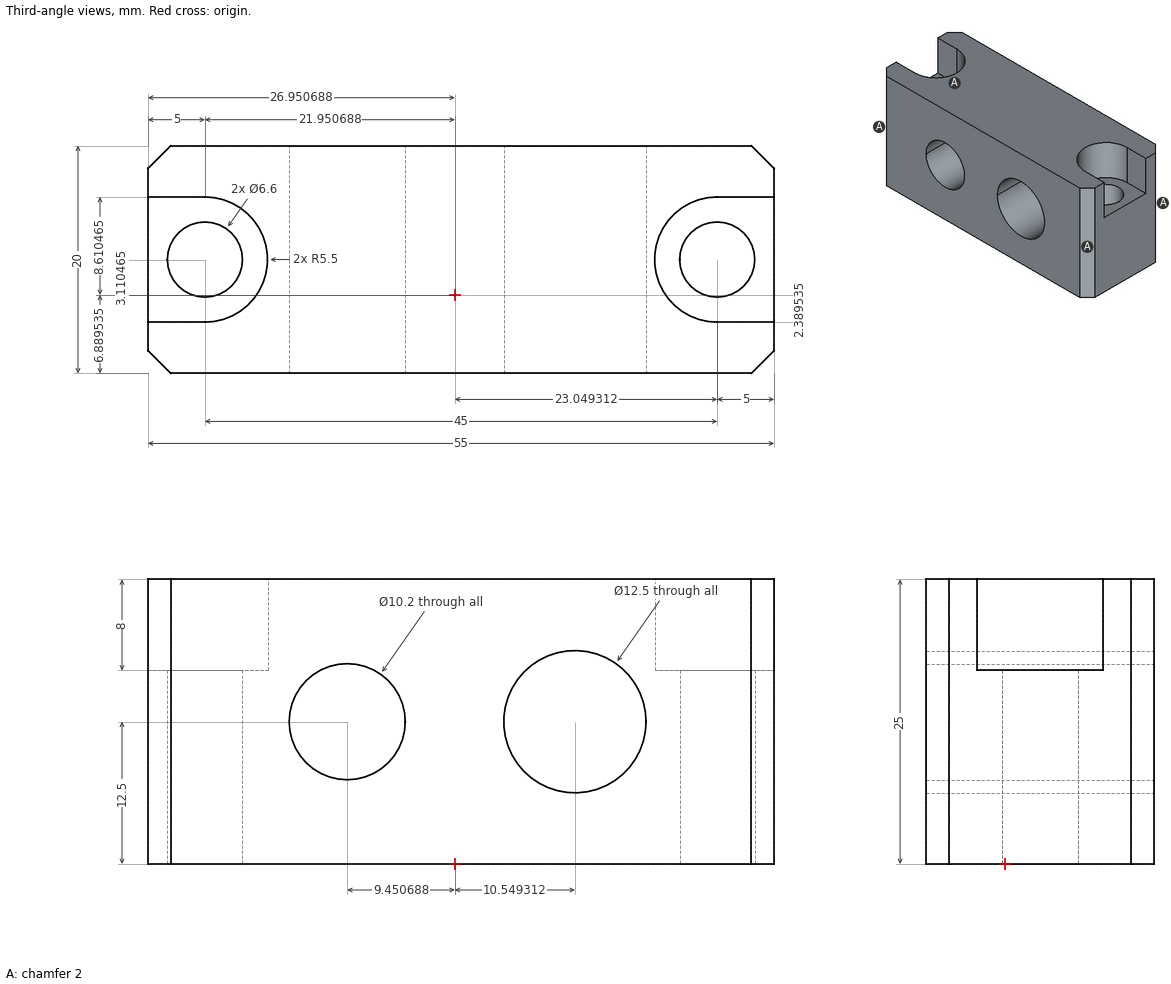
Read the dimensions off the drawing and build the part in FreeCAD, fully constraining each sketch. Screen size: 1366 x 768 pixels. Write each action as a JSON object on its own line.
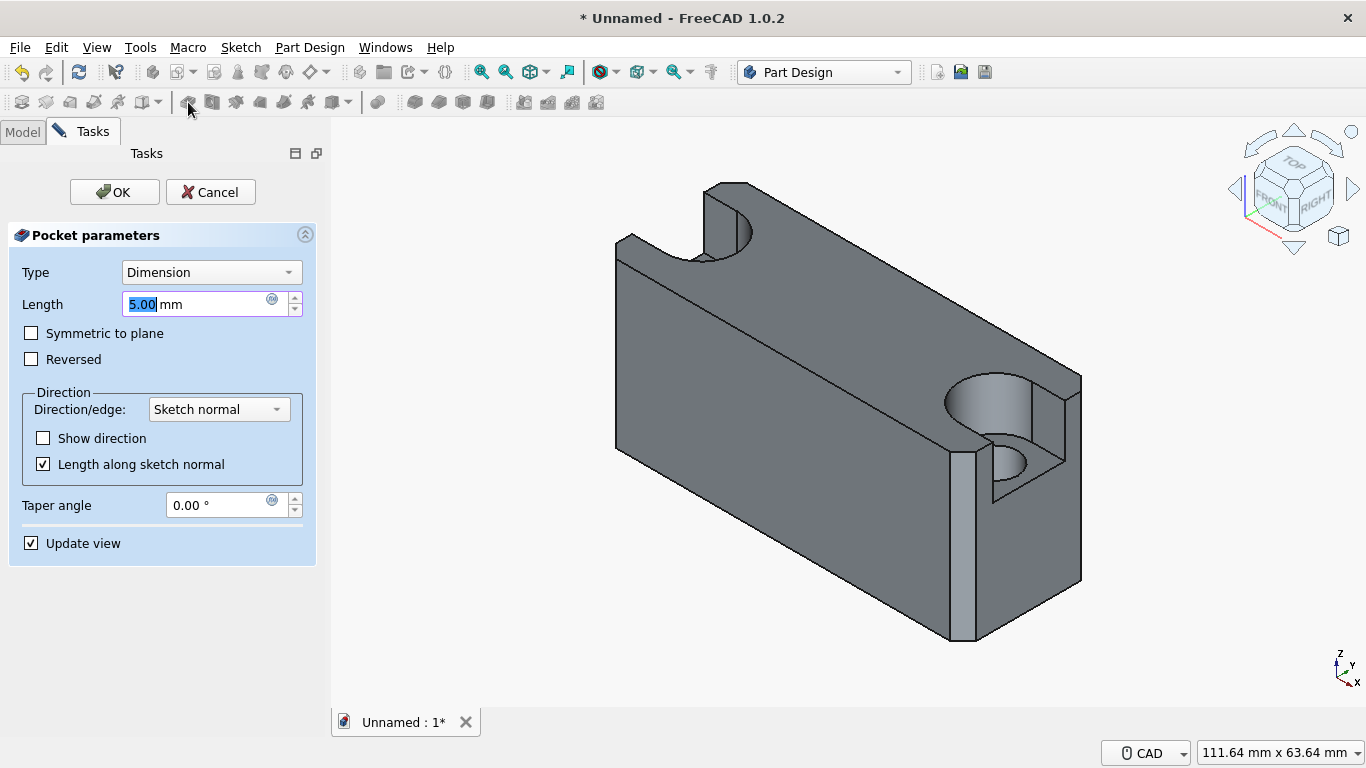
{"action": "left_click", "coordinate": [212, 272]}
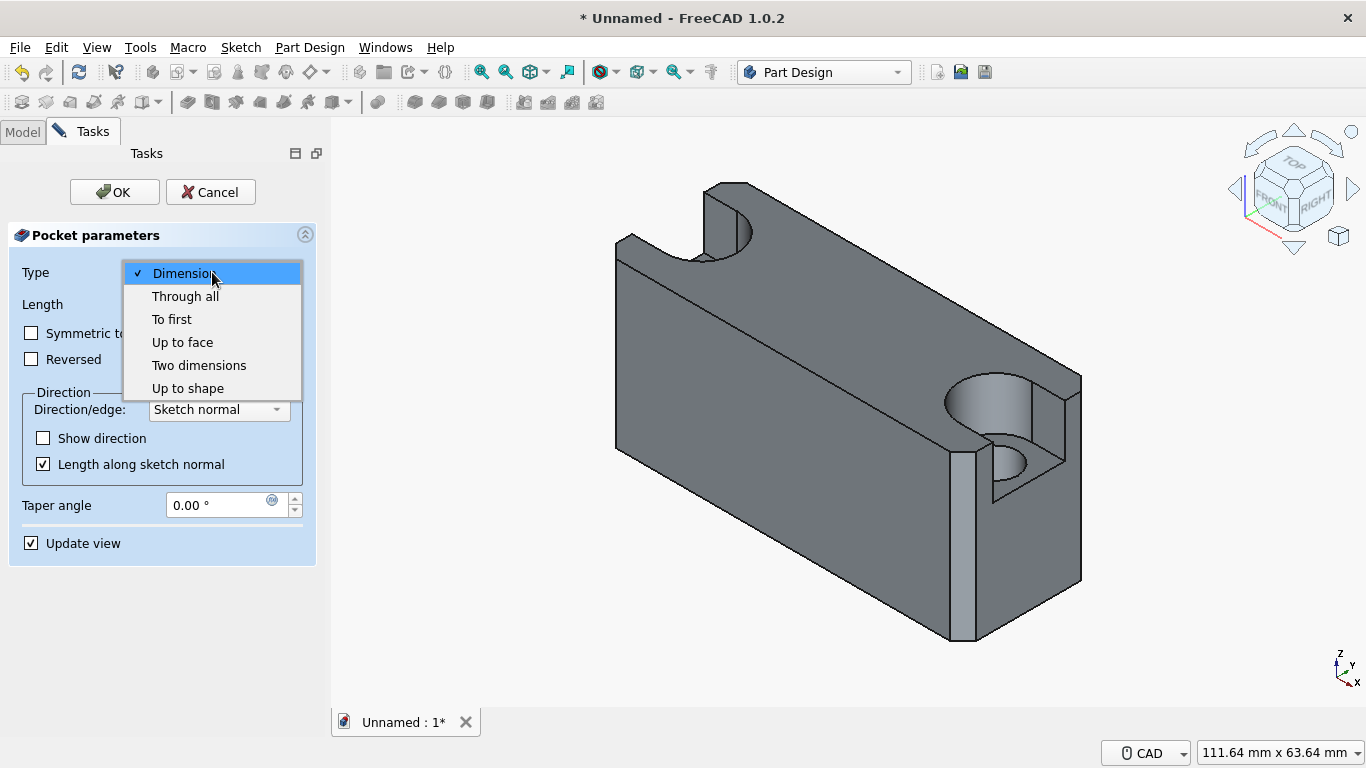
{"action": "left_click", "coordinate": [212, 296]}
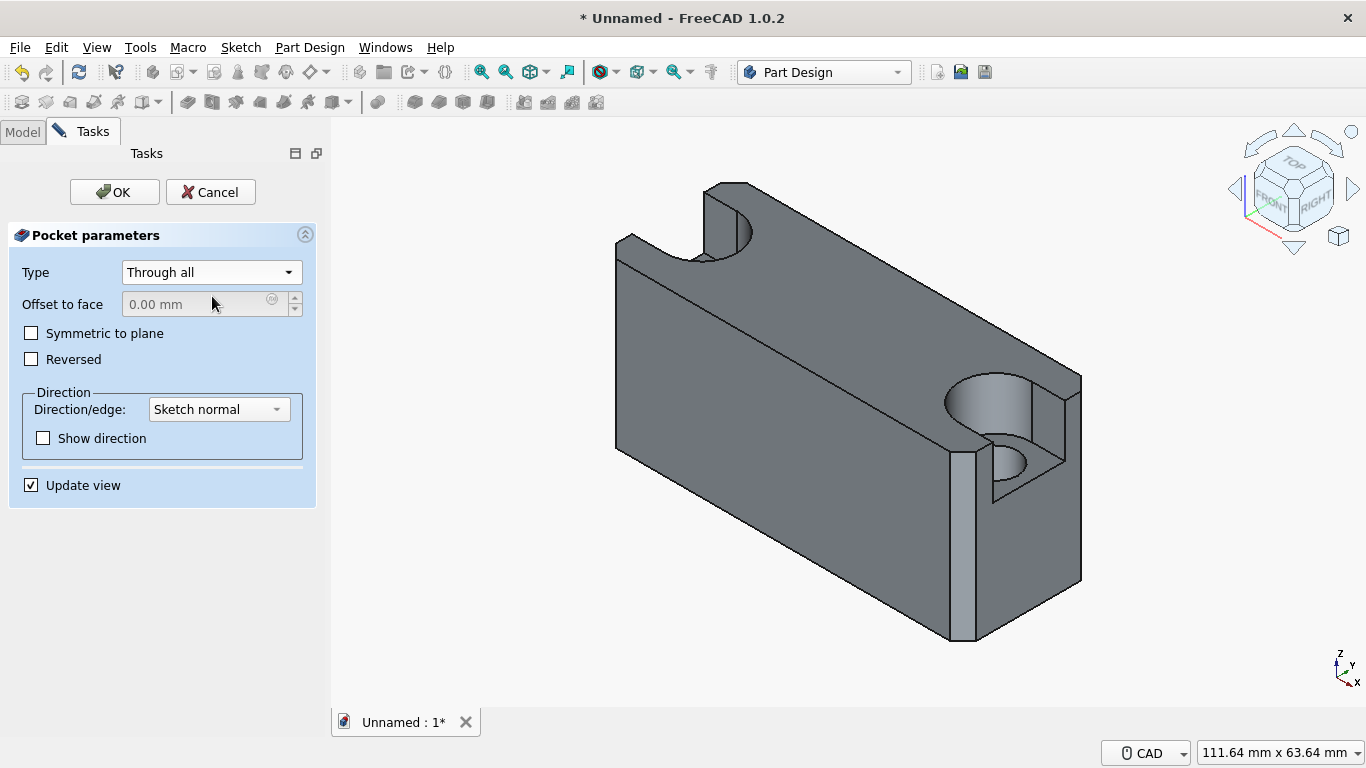
{"action": "left_click", "coordinate": [115, 192]}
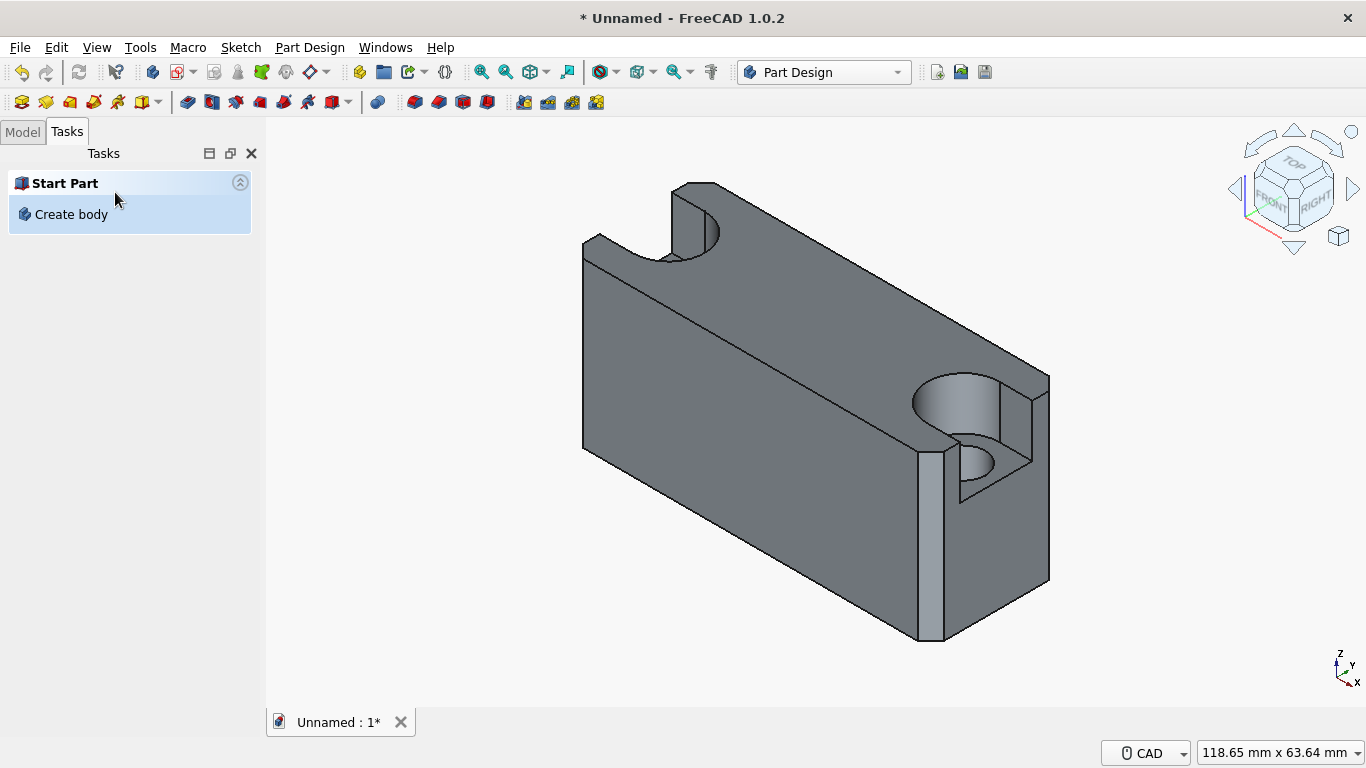
{"action": "left_click", "coordinate": [798, 476]}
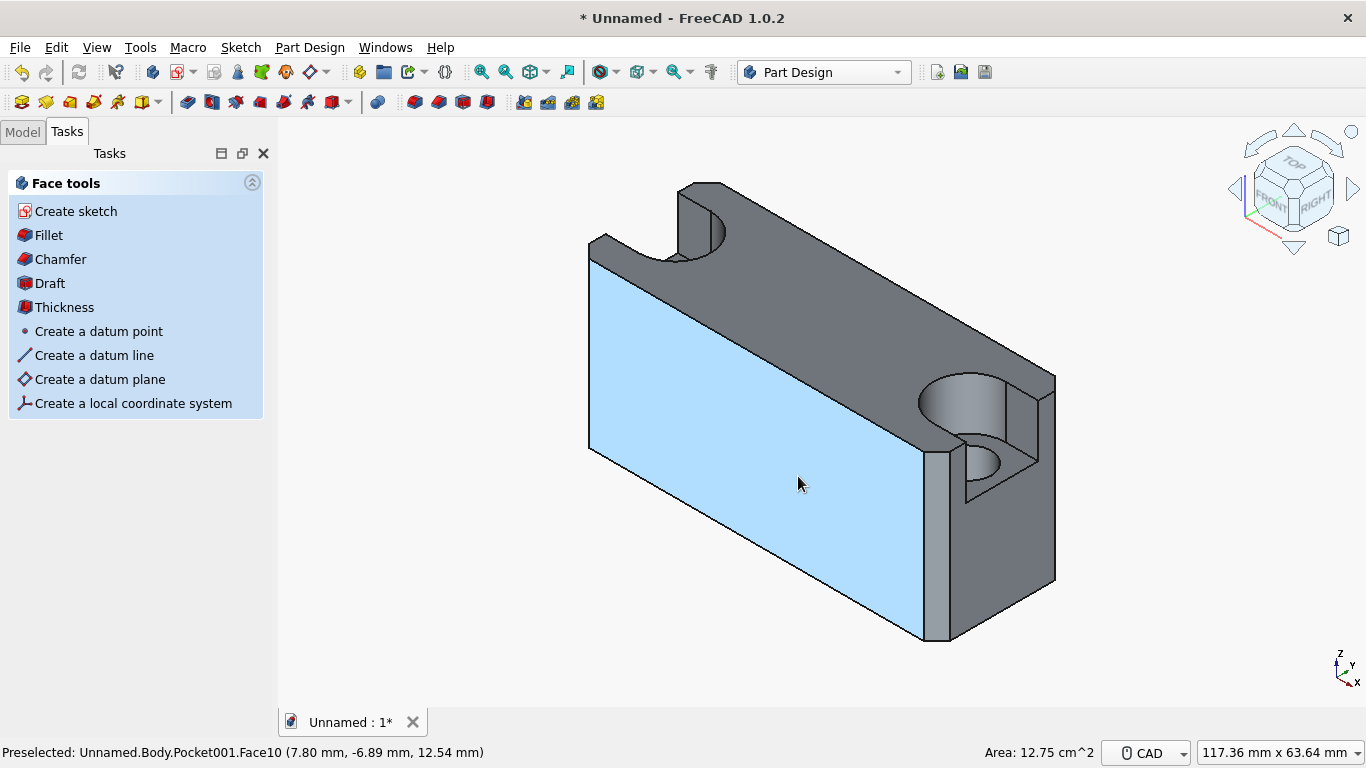
{"action": "left_click", "coordinate": [178, 72]}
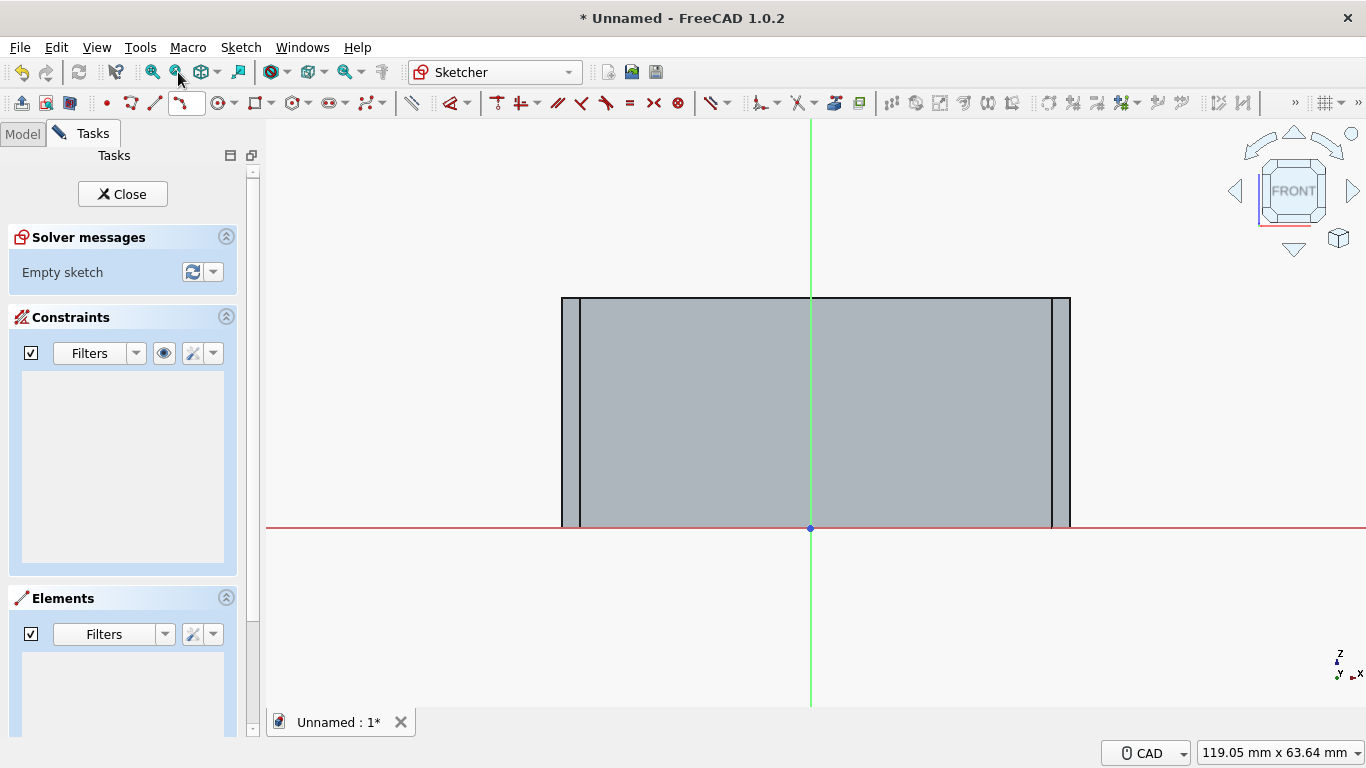
{"action": "scroll", "coordinate": [741, 475], "scroll_direction": "up", "scroll_amount": 4}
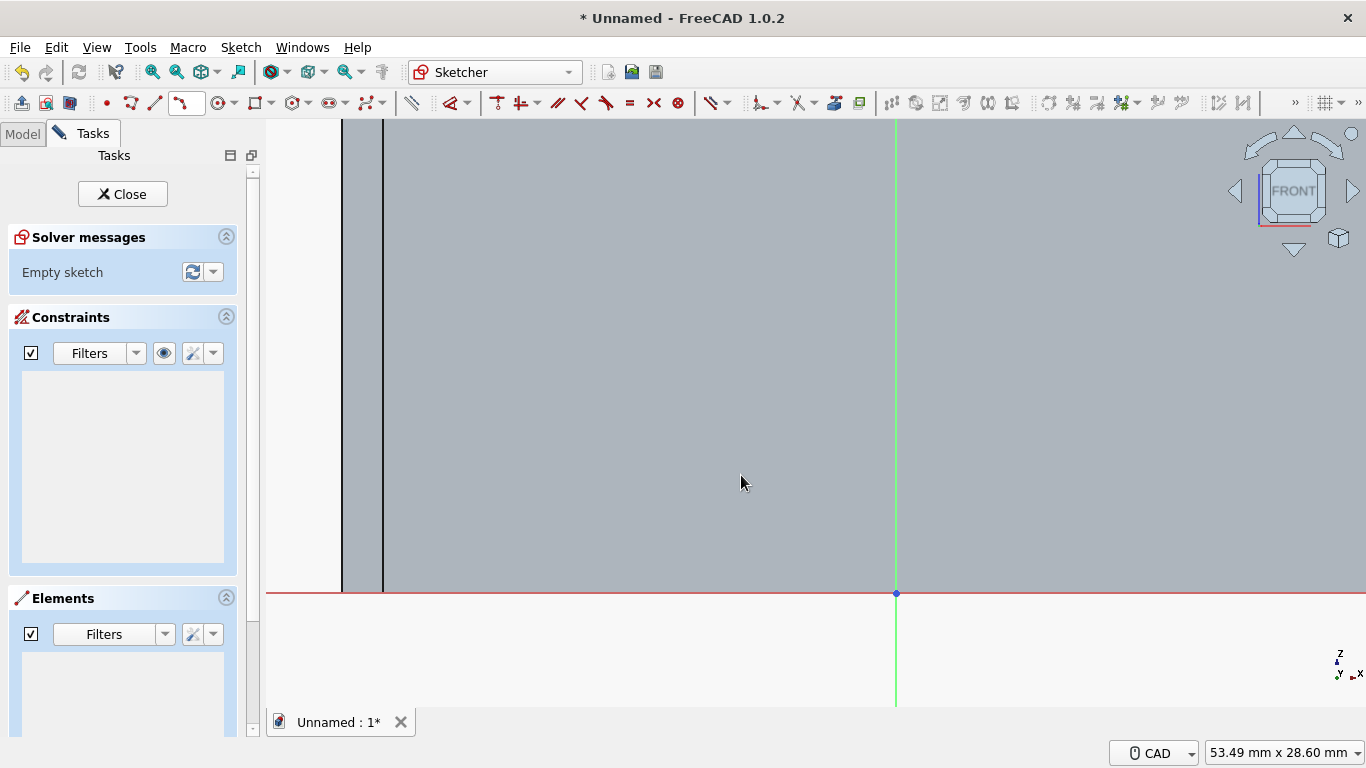
{"action": "left_click", "coordinate": [218, 104]}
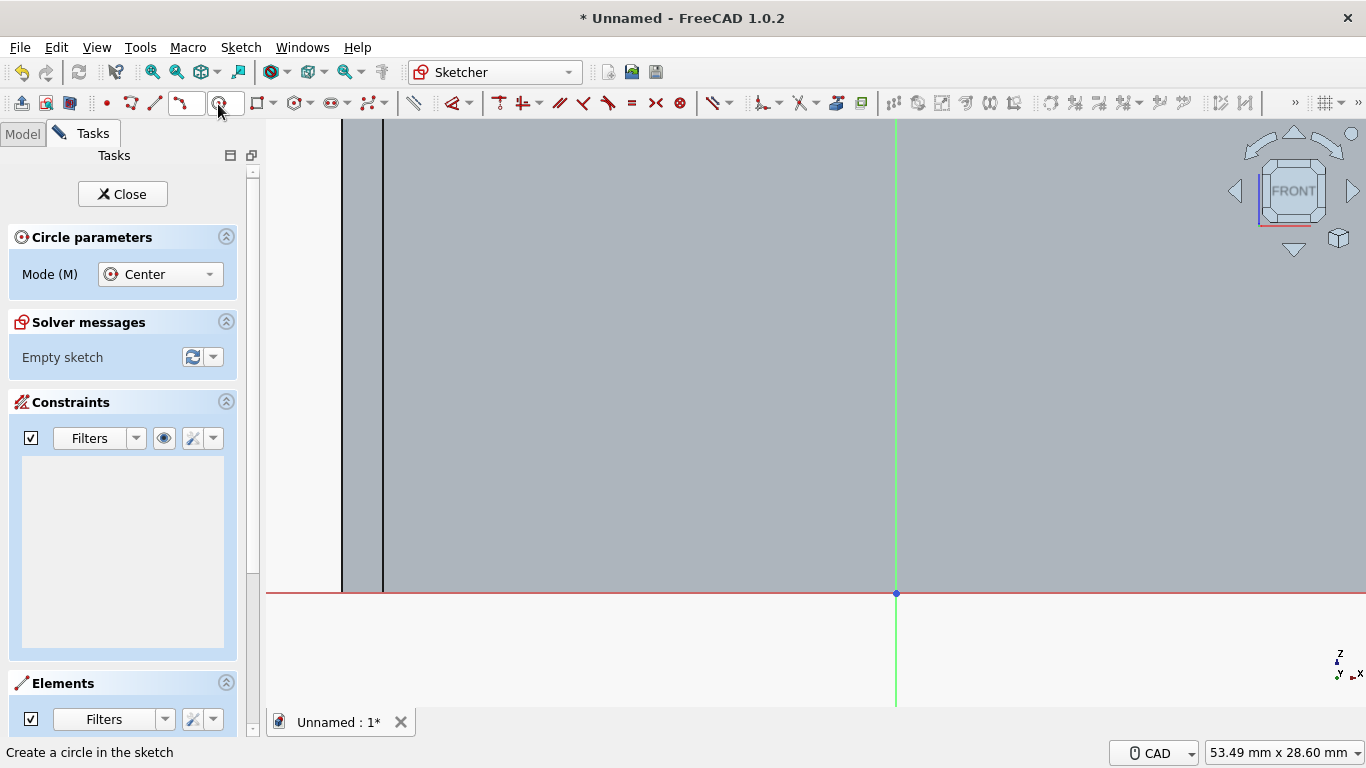
{"action": "left_click", "coordinate": [702, 336]}
{"action": "left_click", "coordinate": [776, 262]}
{"action": "key", "text": "Escape"}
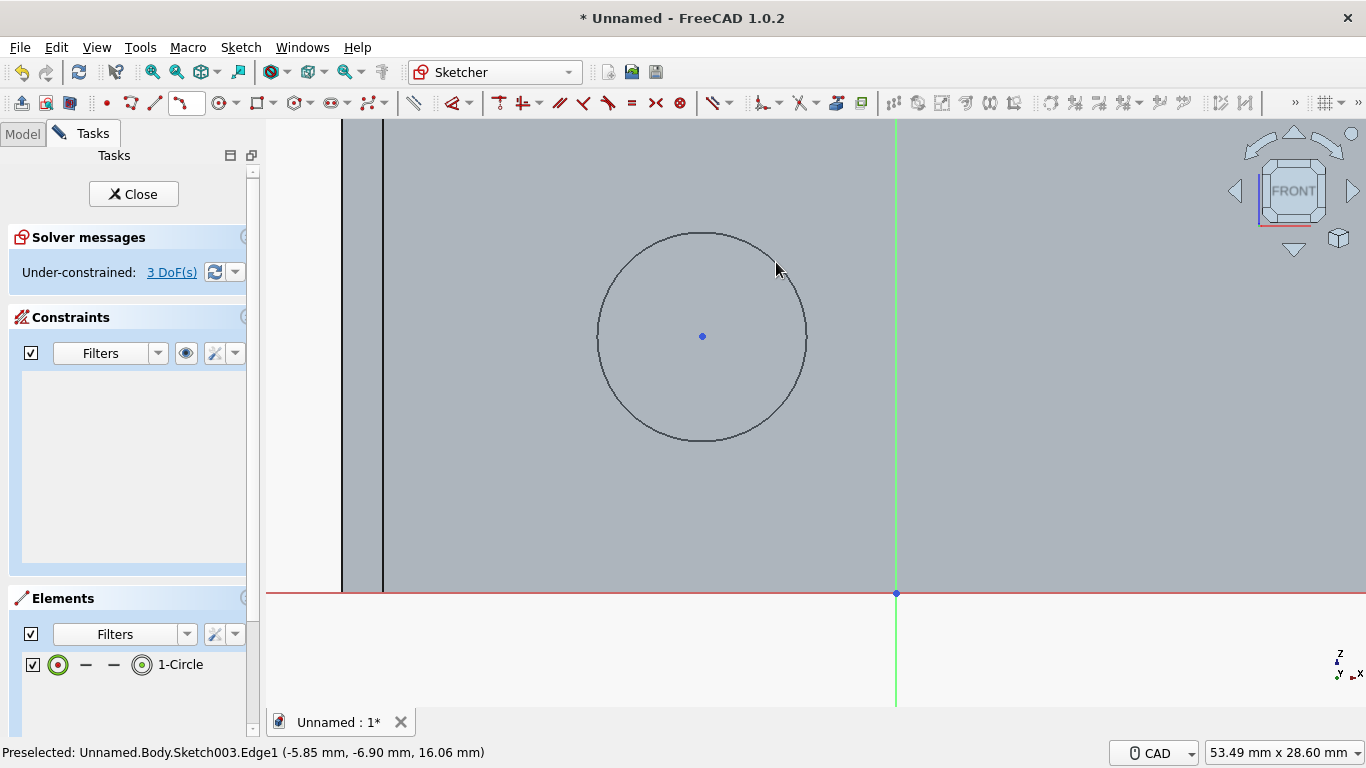
{"action": "key", "text": "d"}